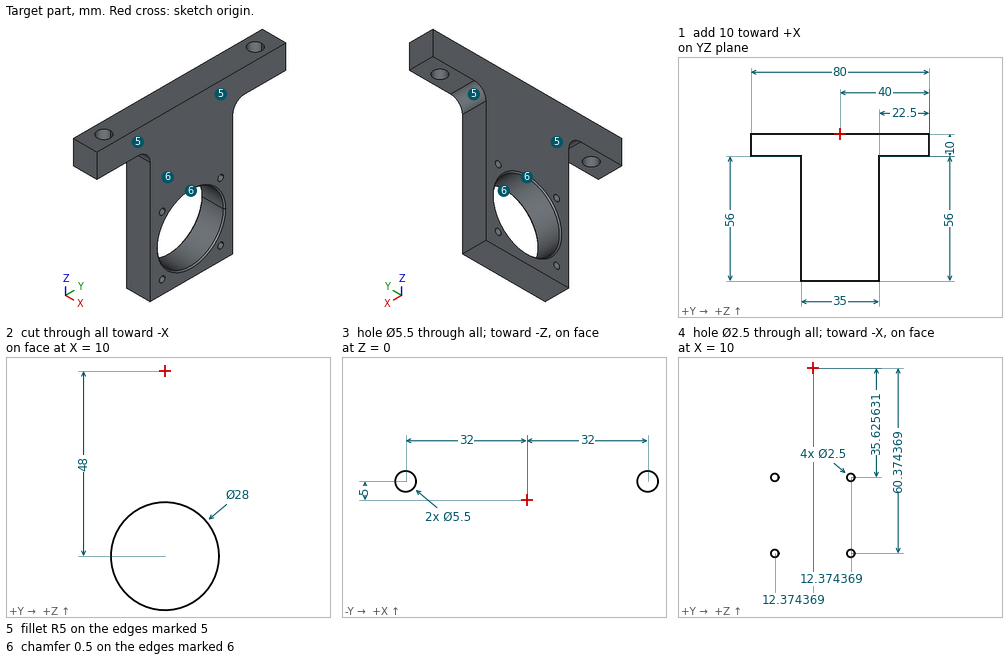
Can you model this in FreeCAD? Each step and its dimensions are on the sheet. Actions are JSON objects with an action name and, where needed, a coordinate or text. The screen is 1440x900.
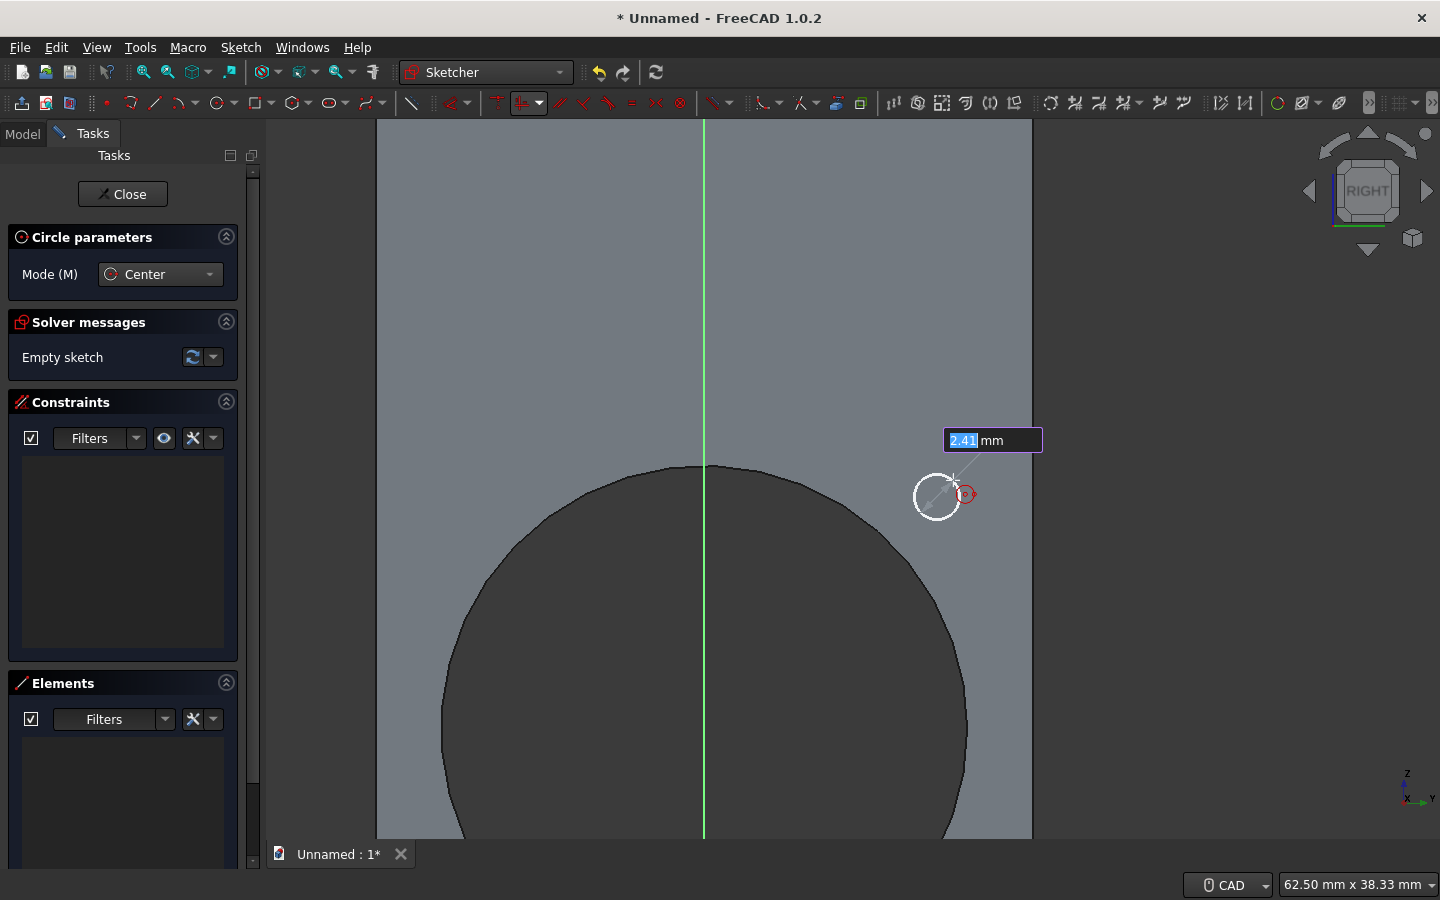
{"action": "type", "text": "2.5"}
{"action": "key", "text": "Return"}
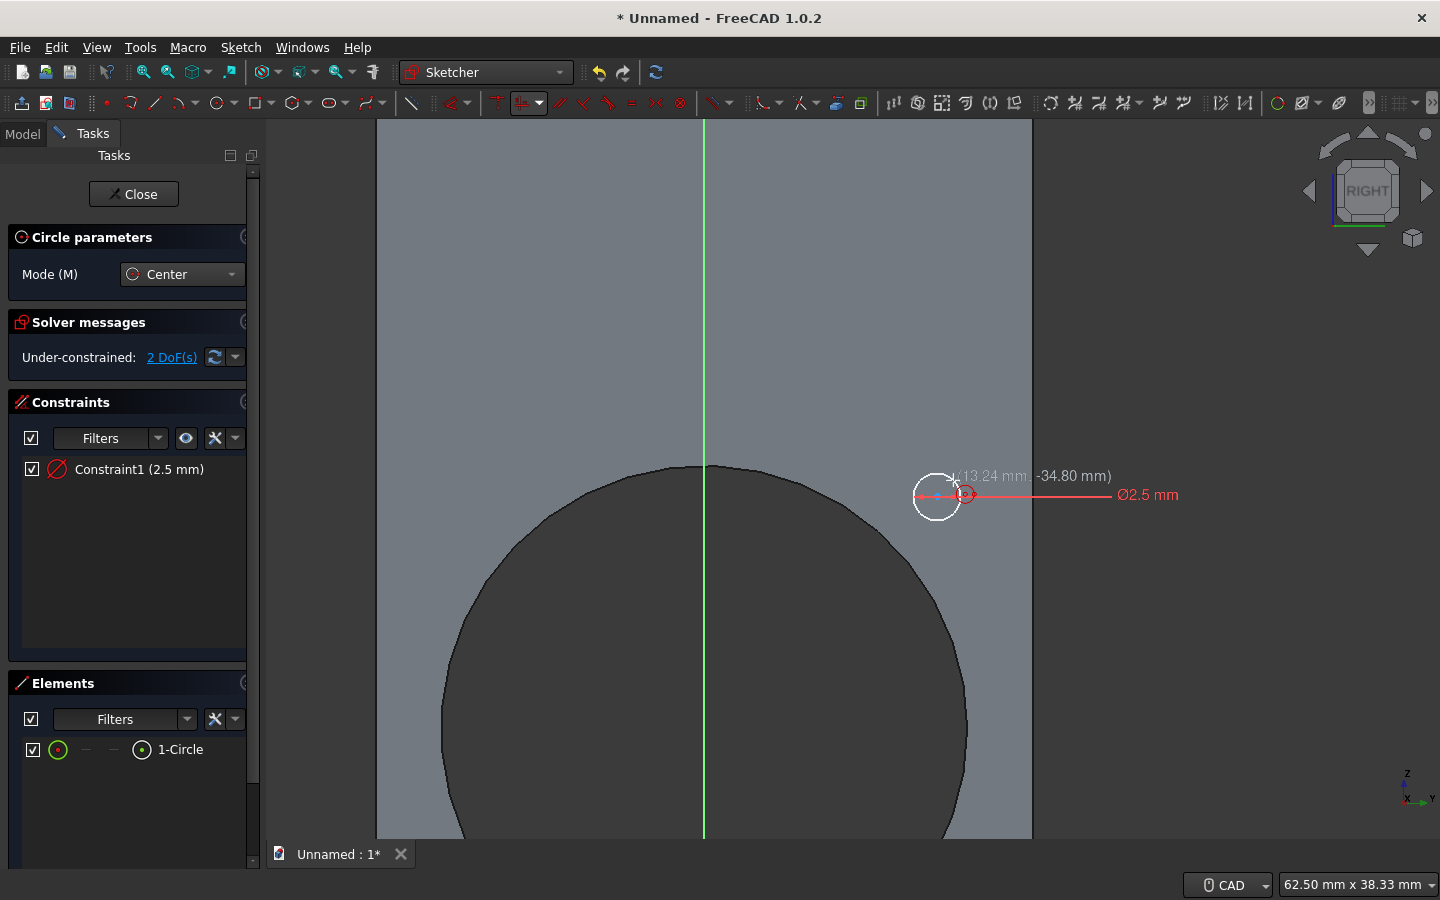
{"action": "scroll", "coordinate": [831, 521], "scroll_direction": "down", "scroll_amount": 5}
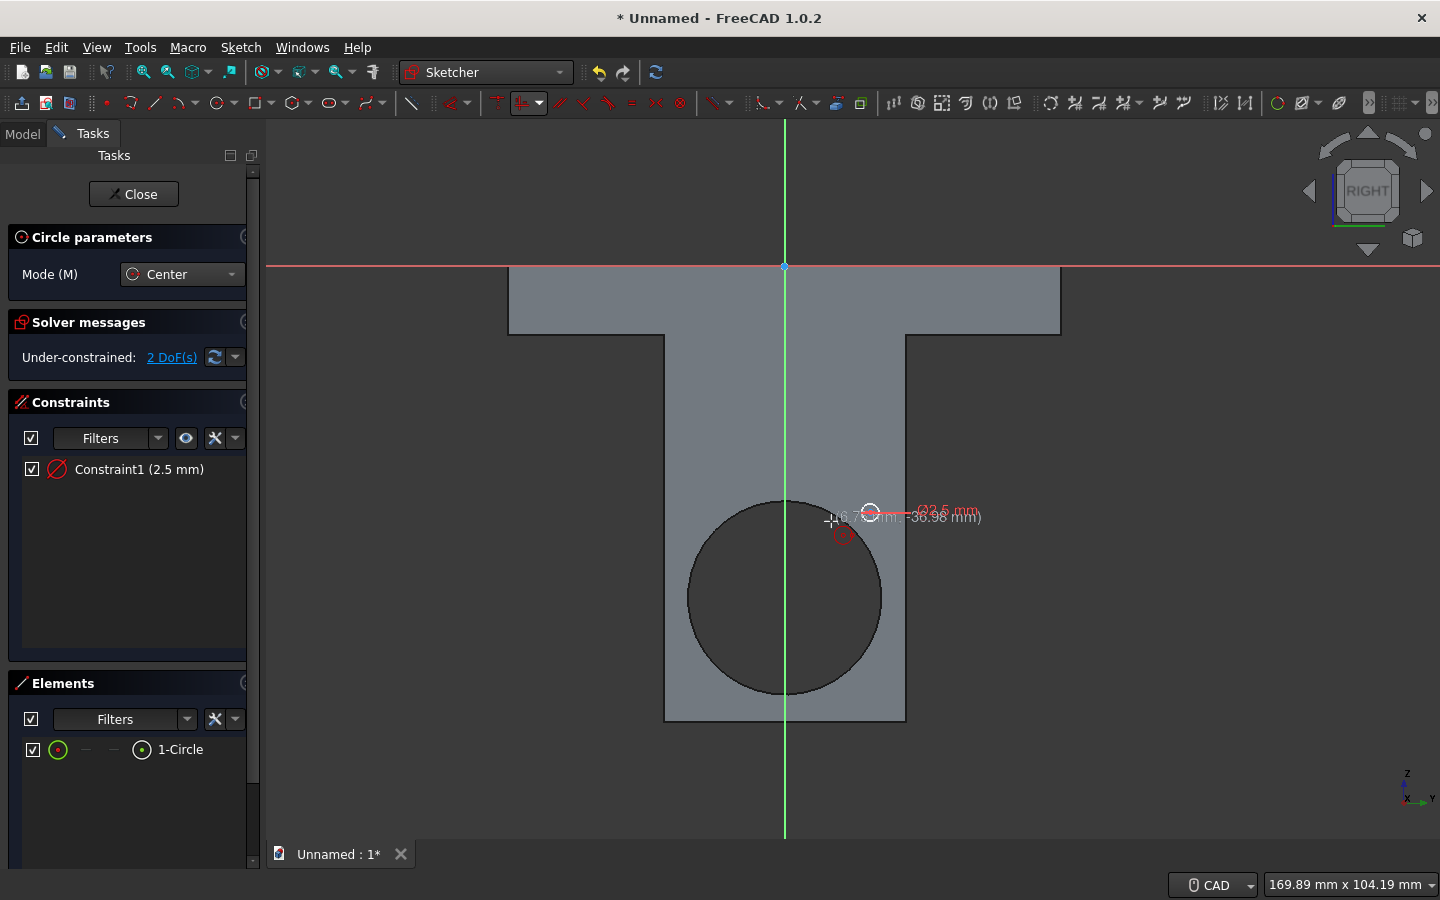
{"action": "scroll", "coordinate": [870, 683], "scroll_direction": "up", "scroll_amount": 5}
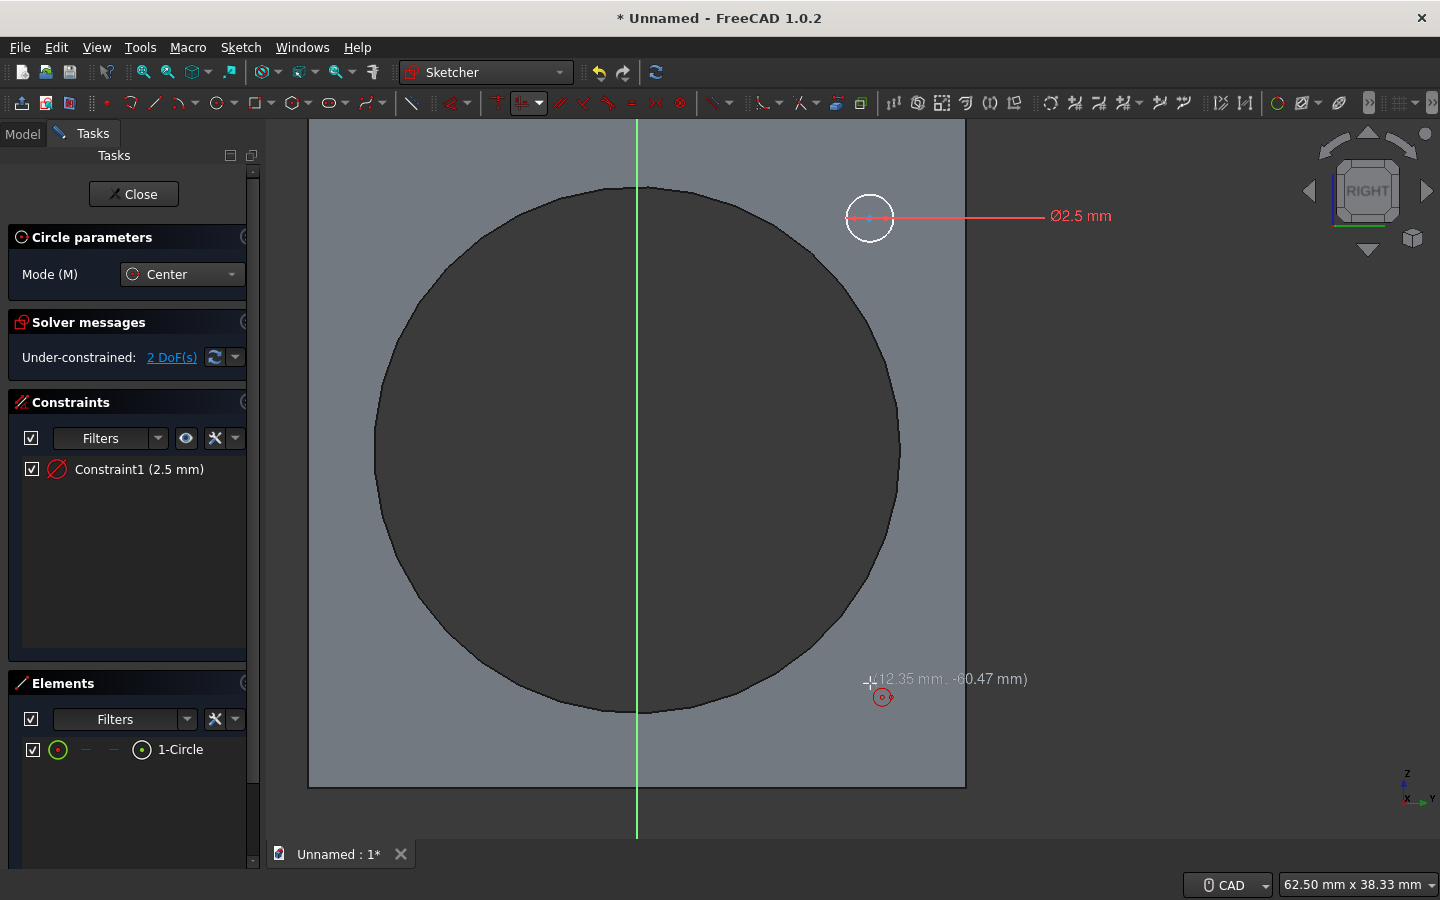
{"action": "left_click", "coordinate": [870, 683]}
{"action": "mouse_move", "coordinate": [886, 666]}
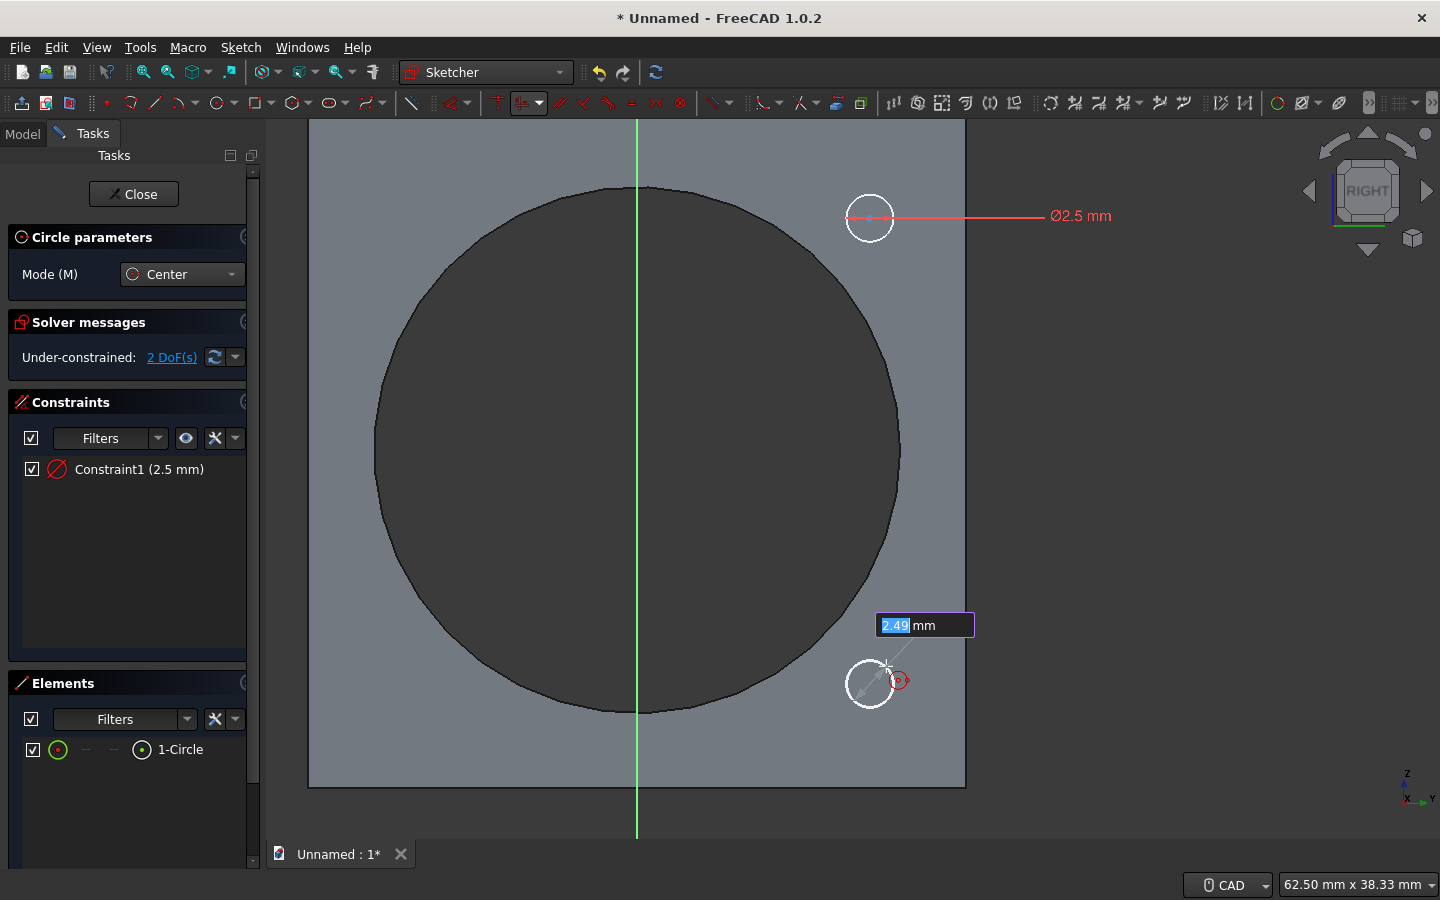
{"action": "type", "text": "2.5"}
{"action": "key", "text": "Return"}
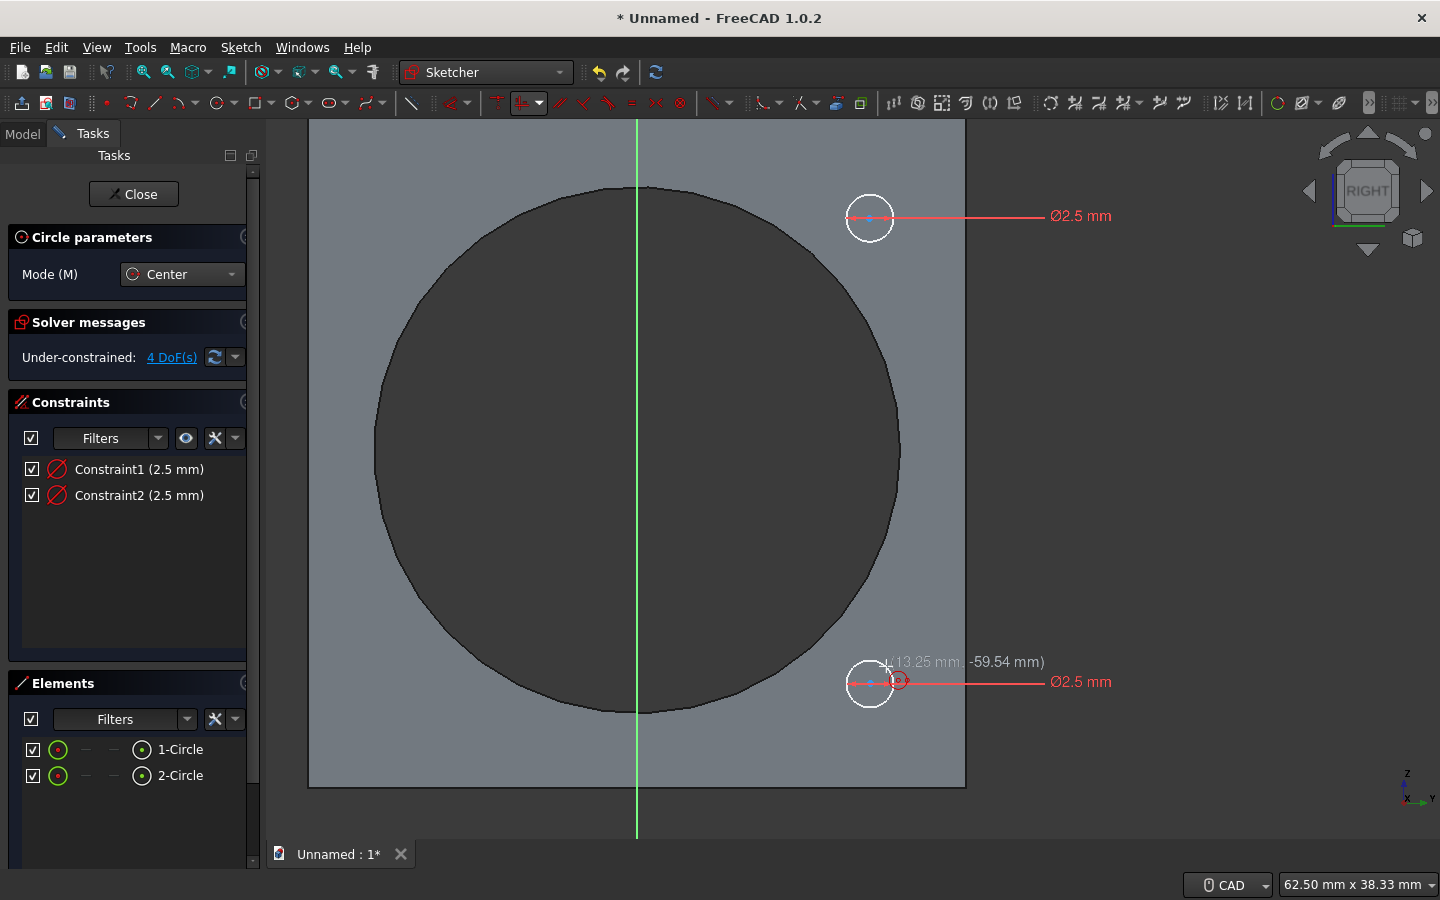
{"action": "left_click", "coordinate": [405, 683]}
{"action": "mouse_move", "coordinate": [421, 666]}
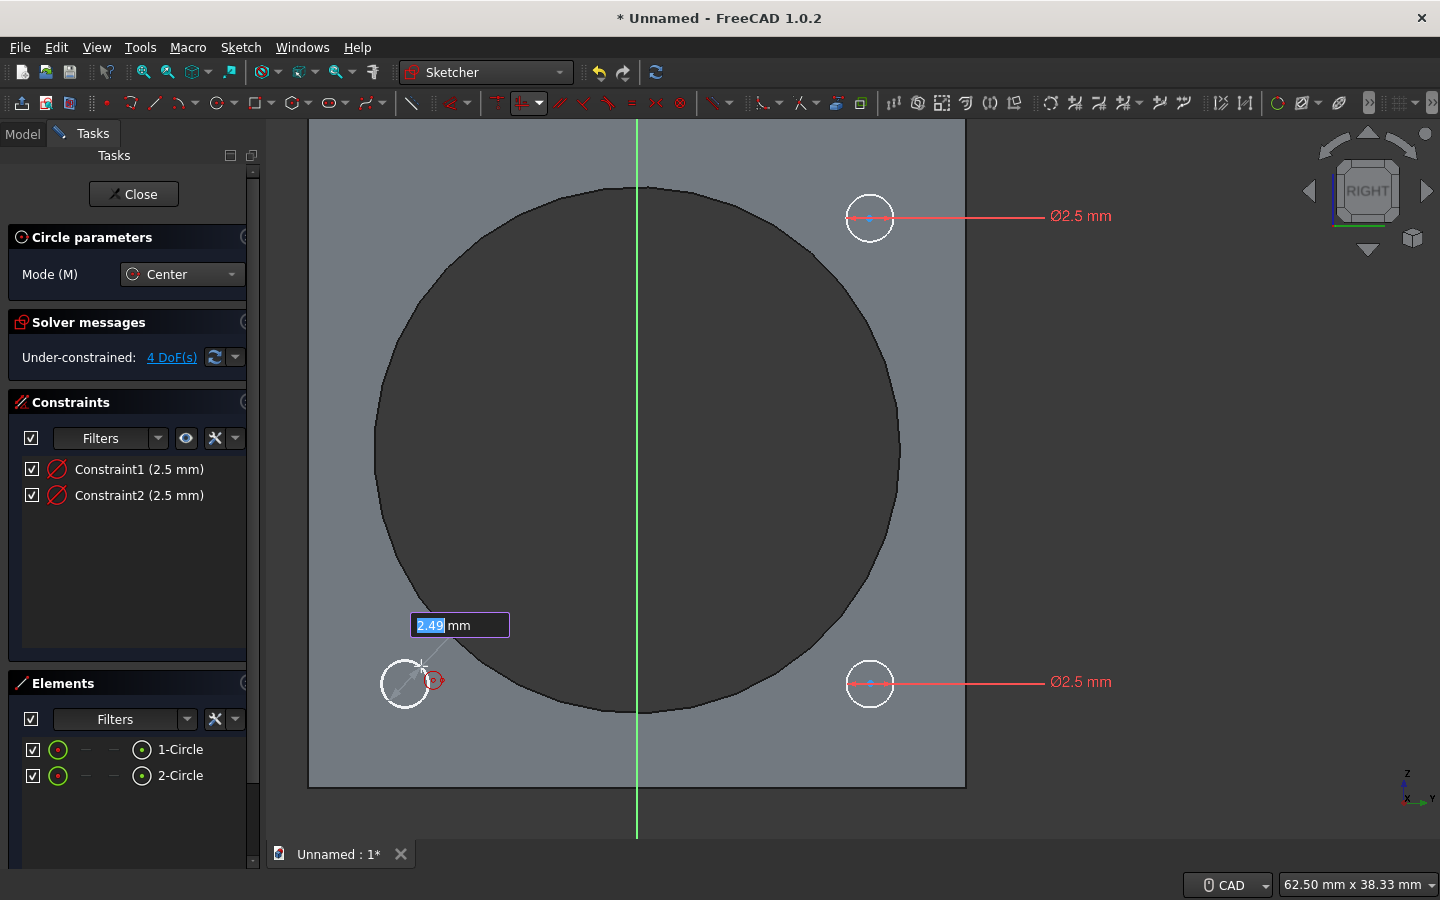
{"action": "type", "text": "2.5"}
{"action": "key", "text": "Return"}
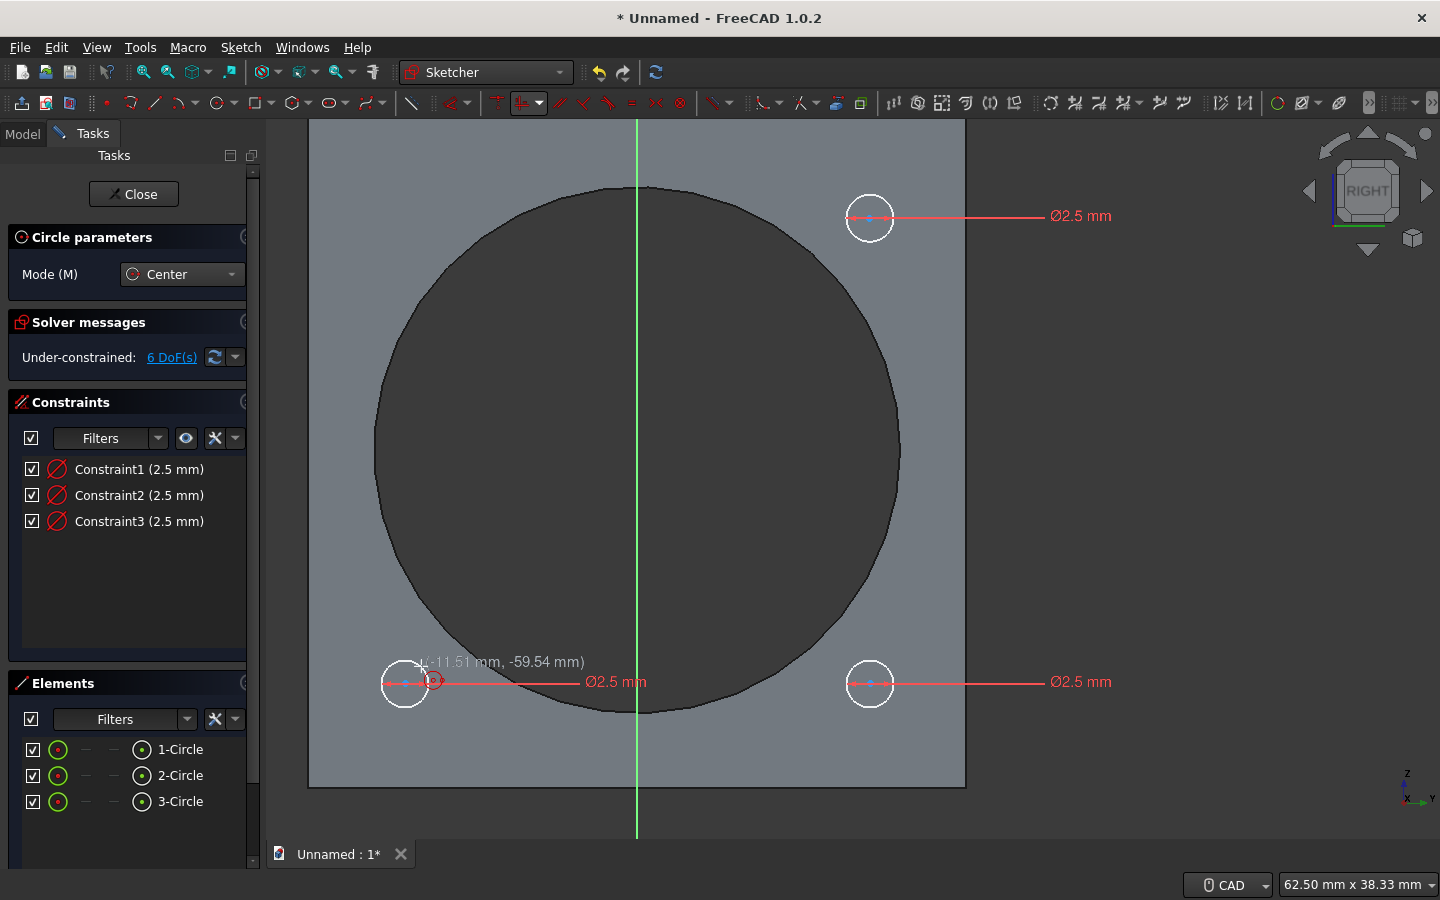
{"action": "left_click", "coordinate": [405, 218]}
{"action": "mouse_move", "coordinate": [421, 201]}